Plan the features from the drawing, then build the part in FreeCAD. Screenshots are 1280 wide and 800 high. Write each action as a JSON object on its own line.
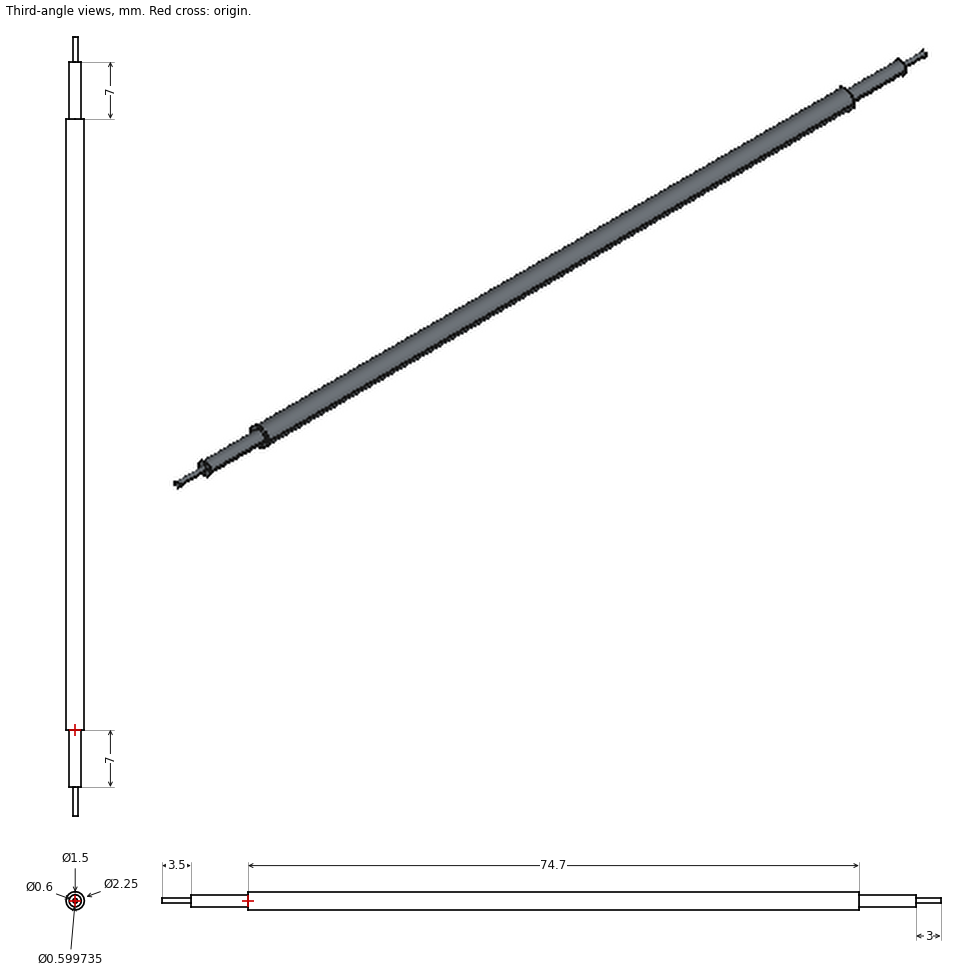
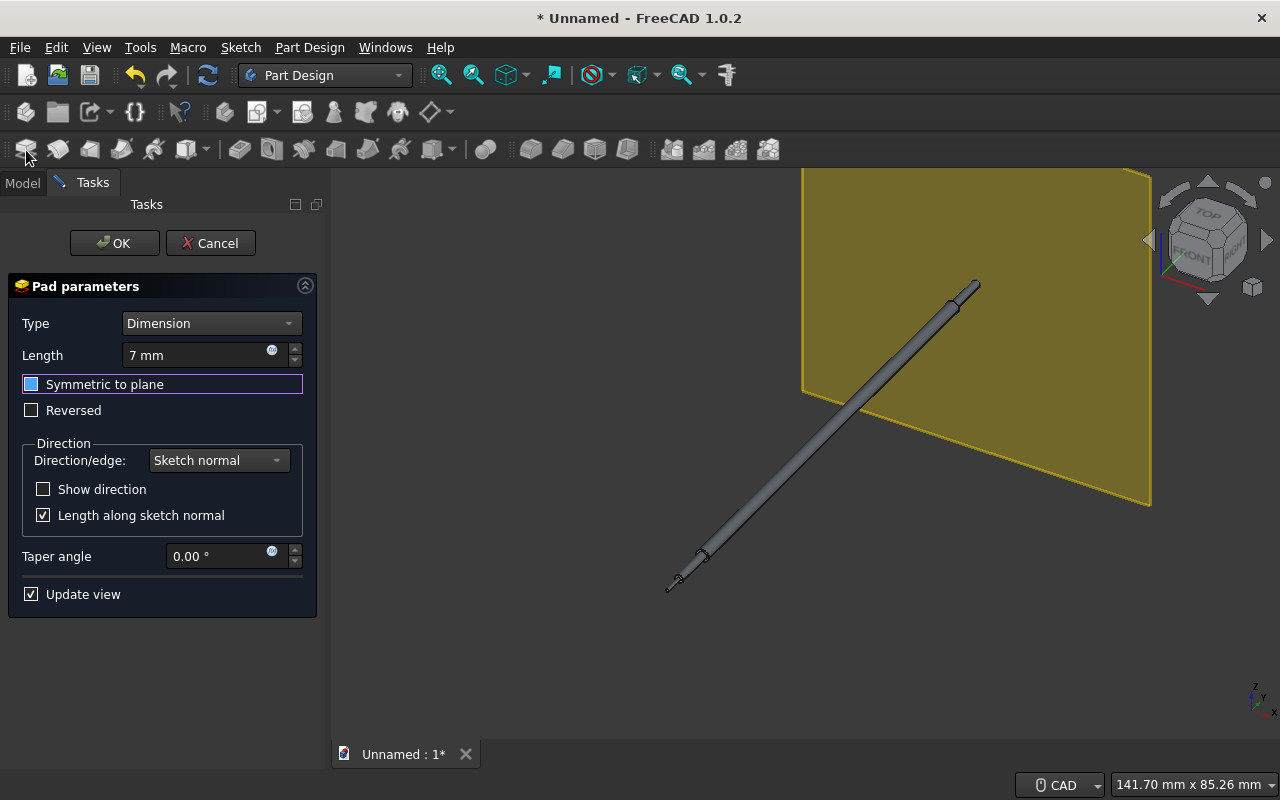
{"action": "left_click", "coordinate": [115, 243]}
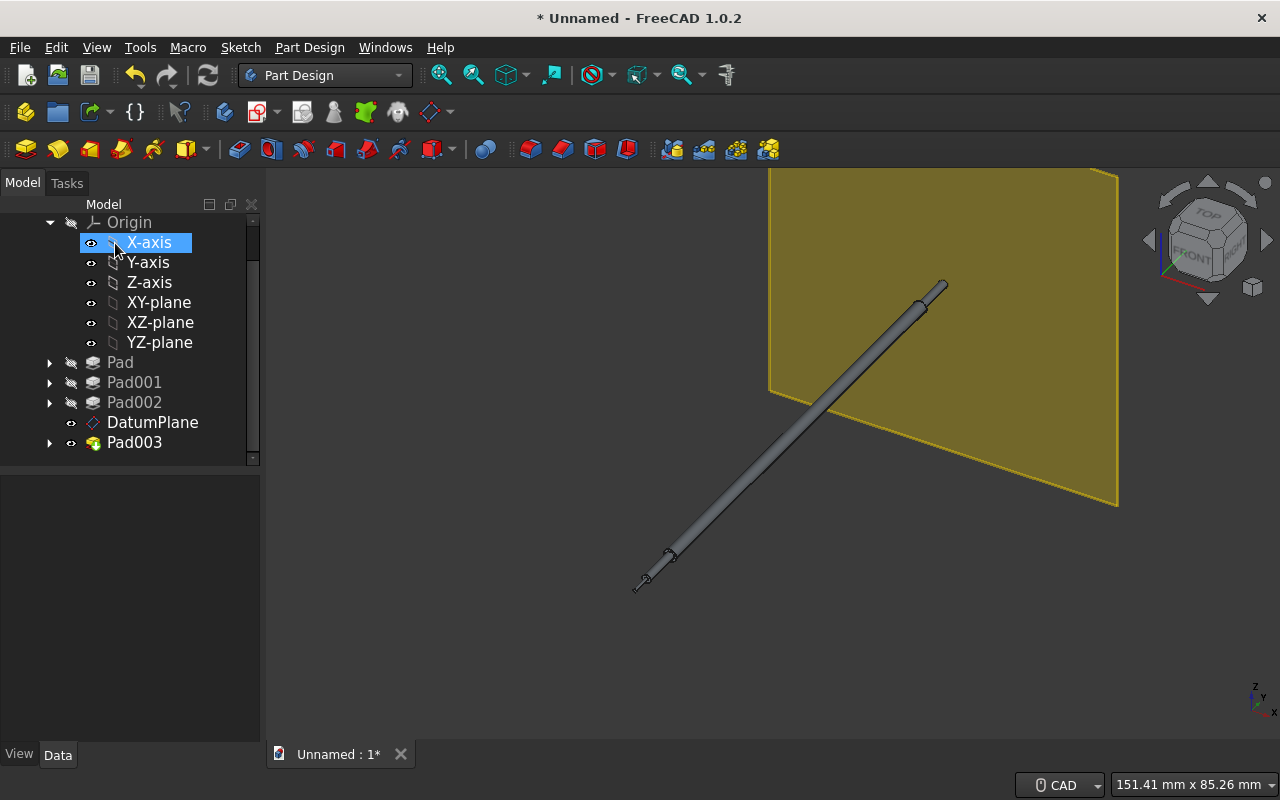
{"action": "left_click", "coordinate": [116, 423]}
{"action": "key", "text": "space"}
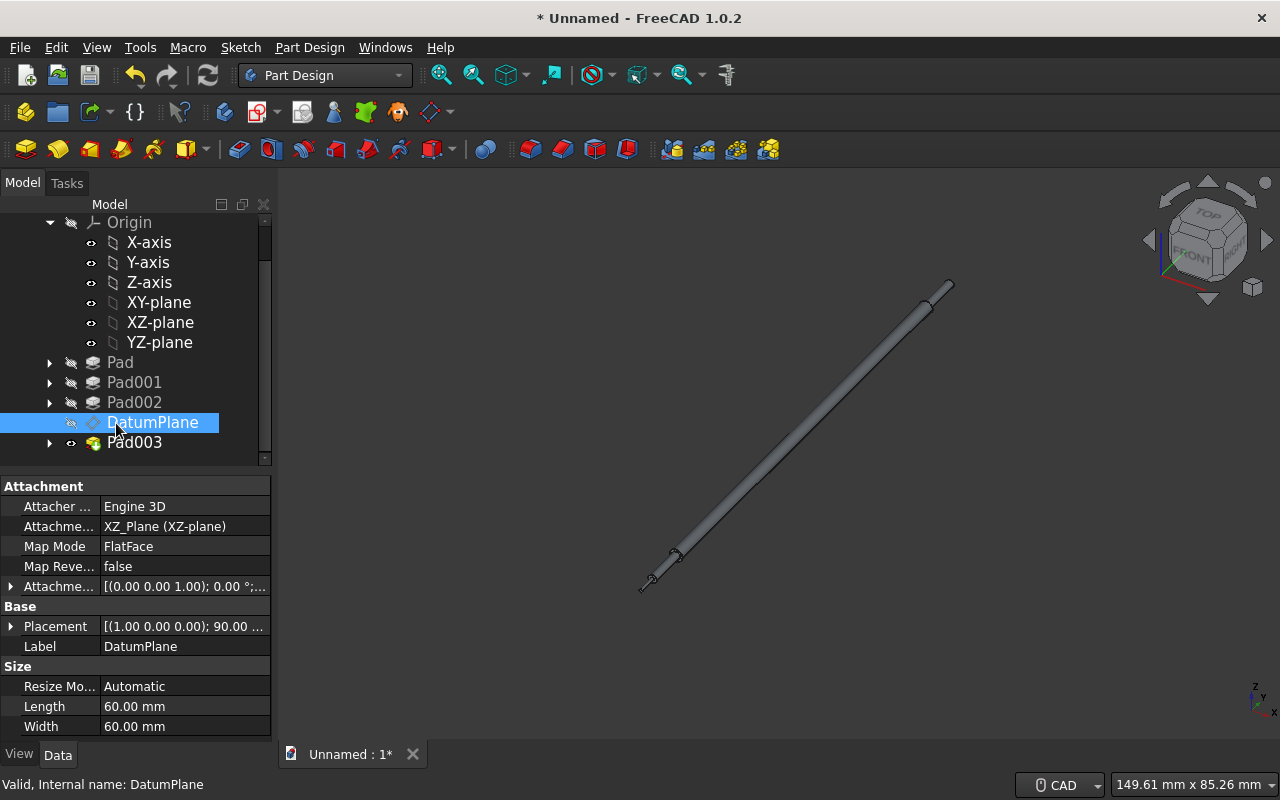
{"action": "key", "text": "4"}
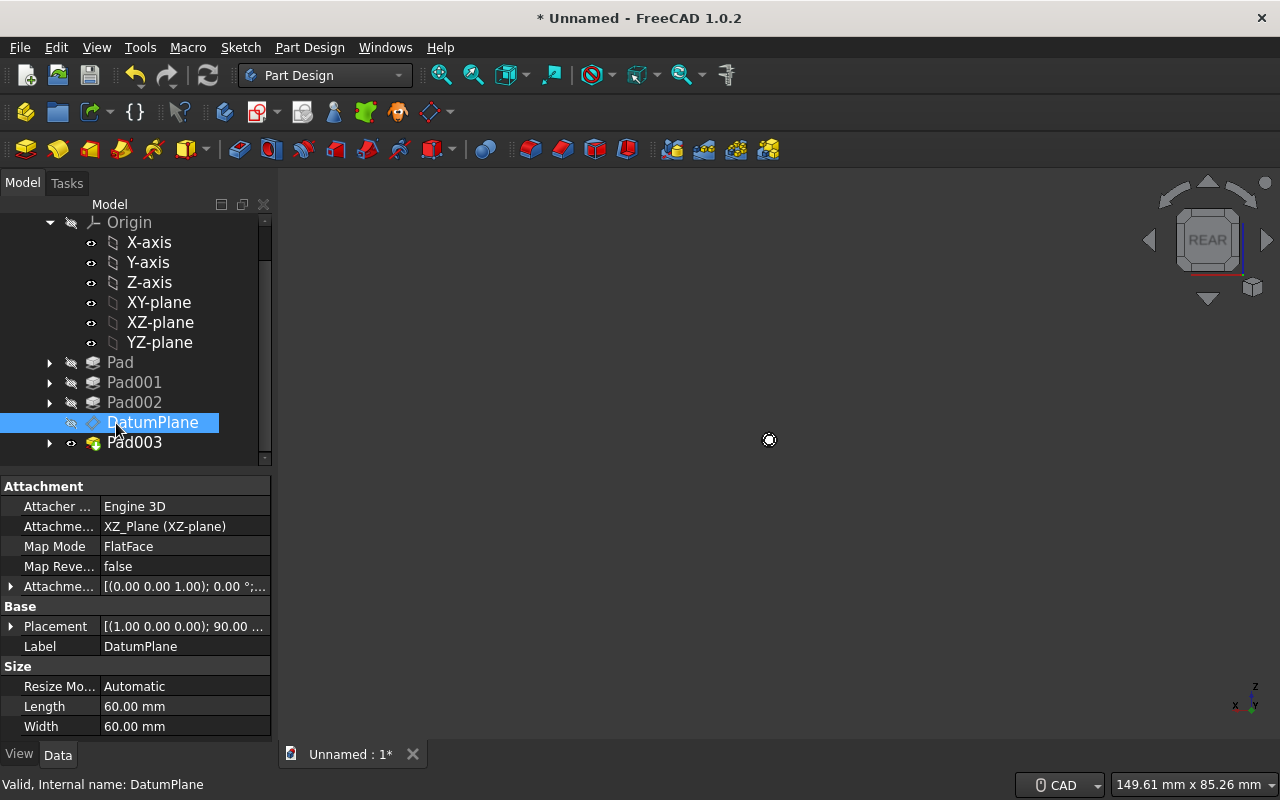
{"action": "left_click", "coordinate": [442, 76]}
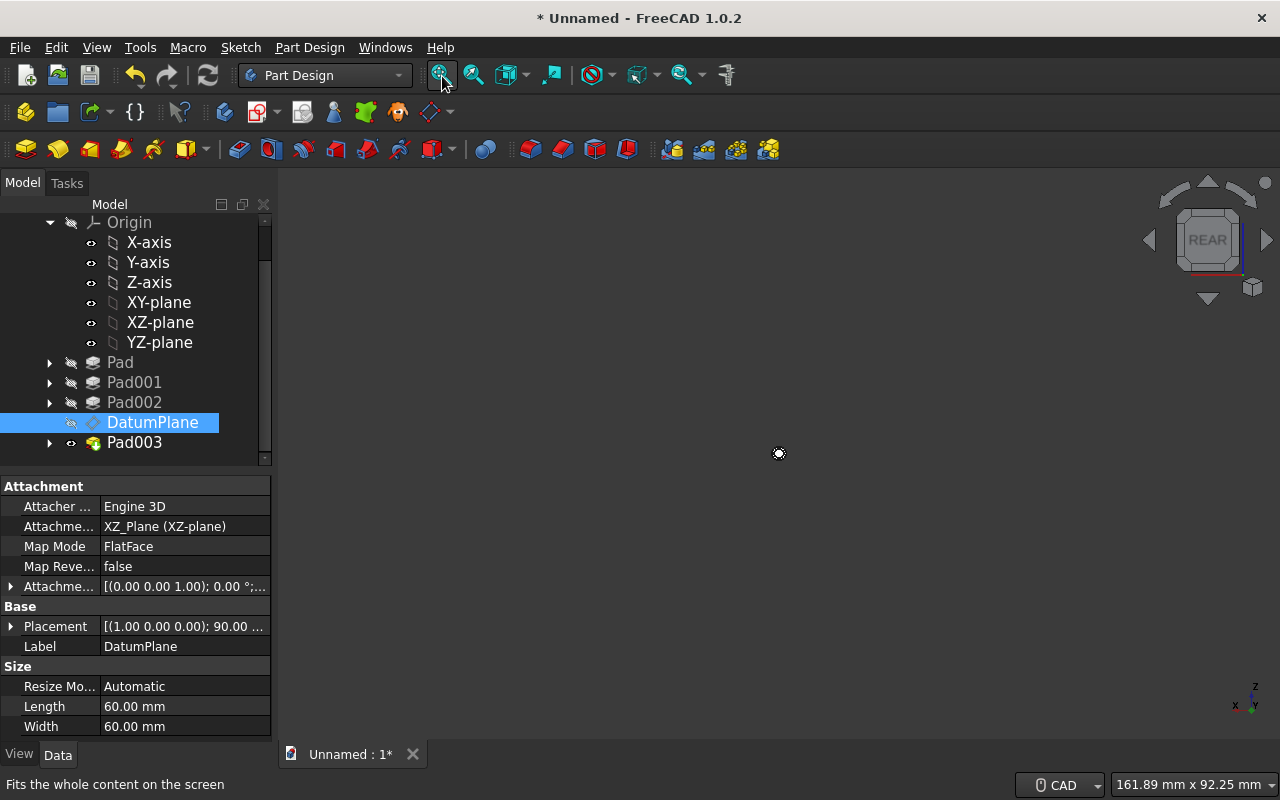
{"action": "scroll", "coordinate": [779, 453], "scroll_direction": "up", "scroll_amount": 5}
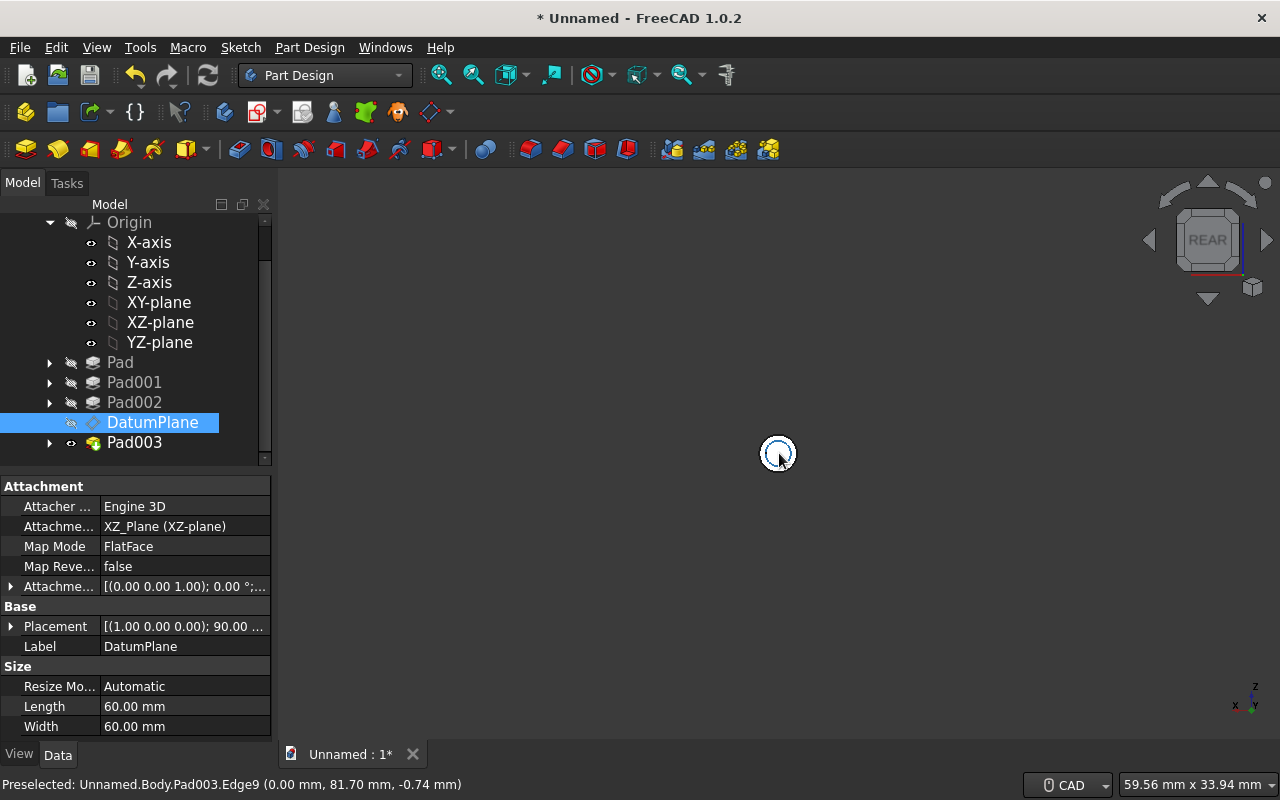
{"action": "left_click", "coordinate": [778, 453]}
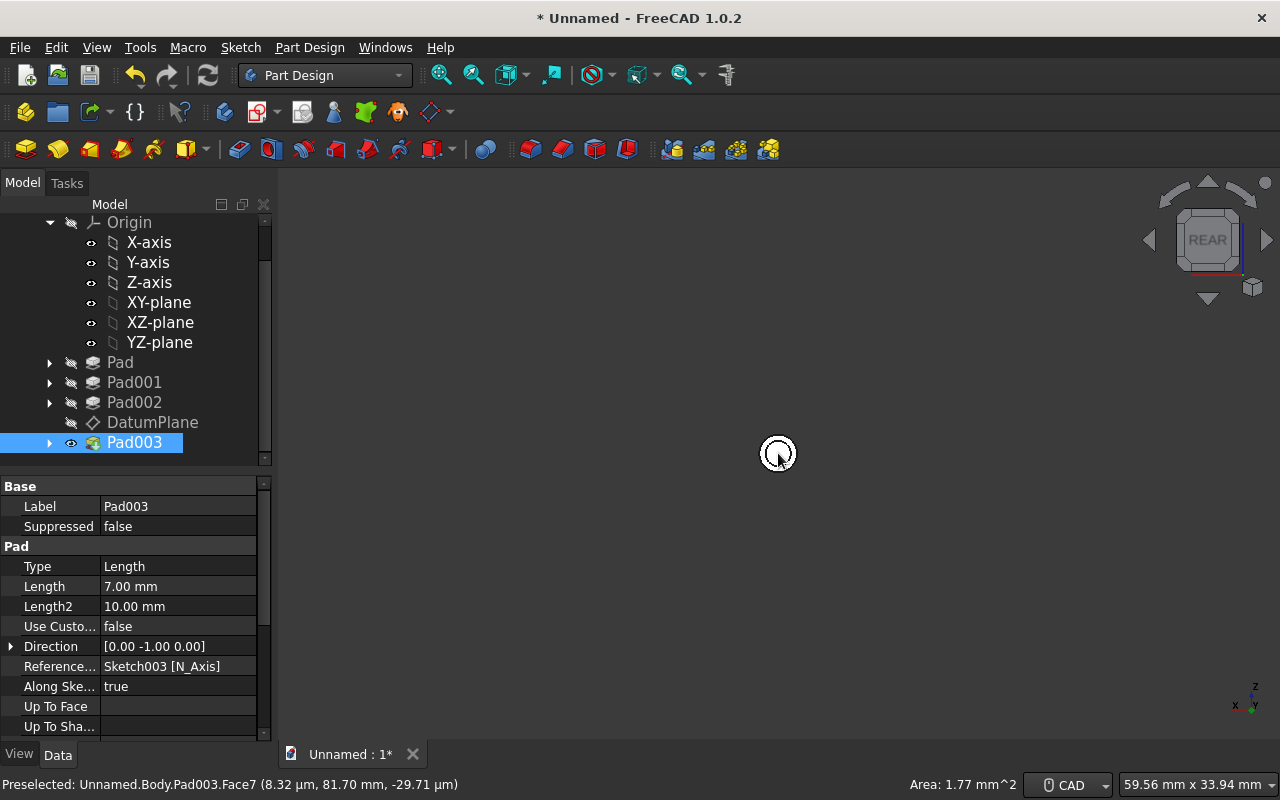
{"action": "left_click", "coordinate": [258, 112]}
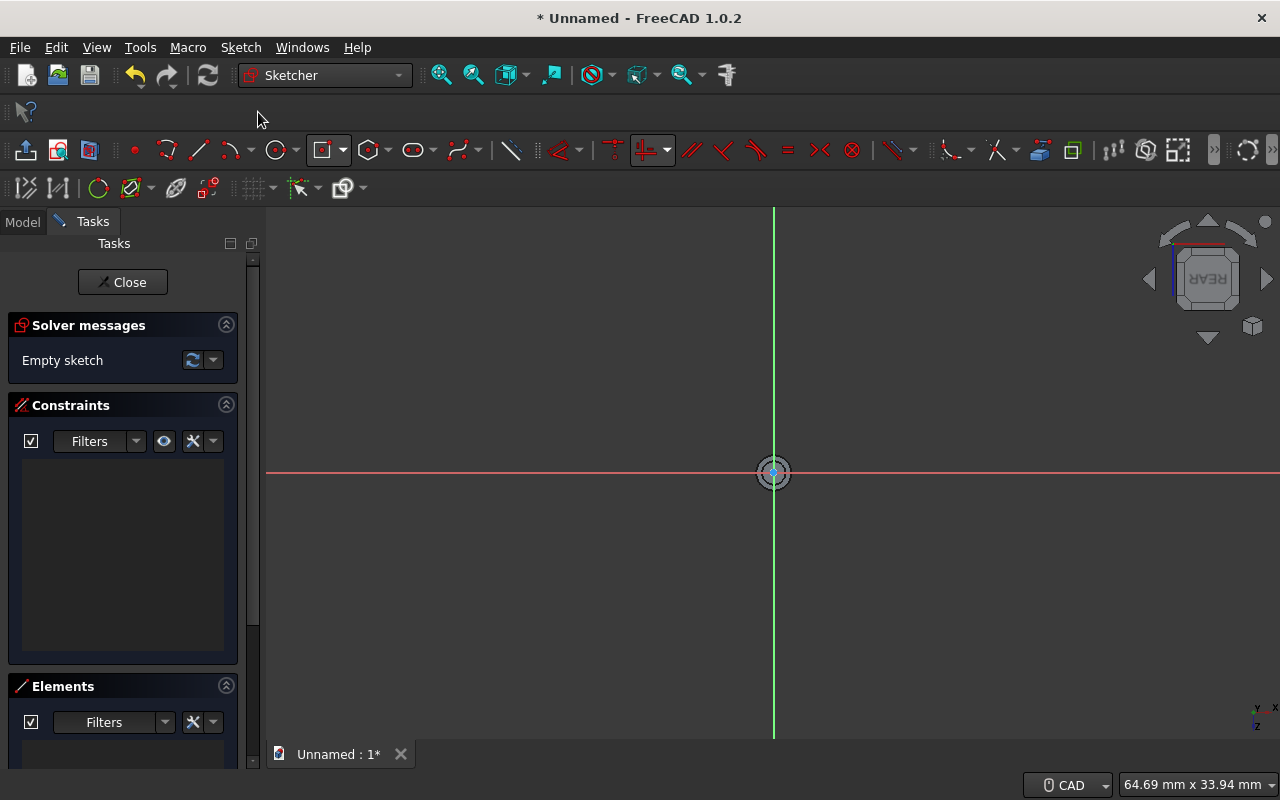
{"action": "scroll", "coordinate": [777, 473], "scroll_direction": "up", "scroll_amount": 15}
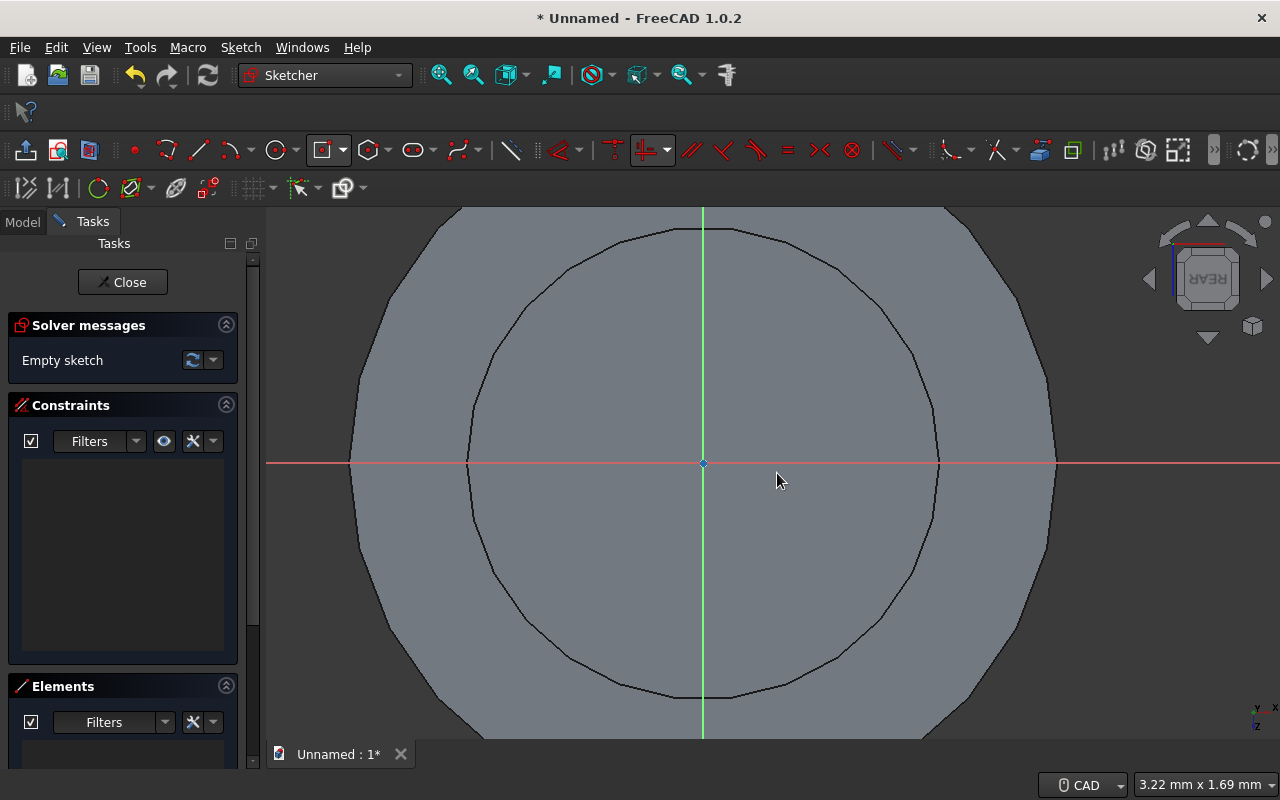
{"action": "scroll", "coordinate": [701, 452], "scroll_direction": "up", "scroll_amount": 3}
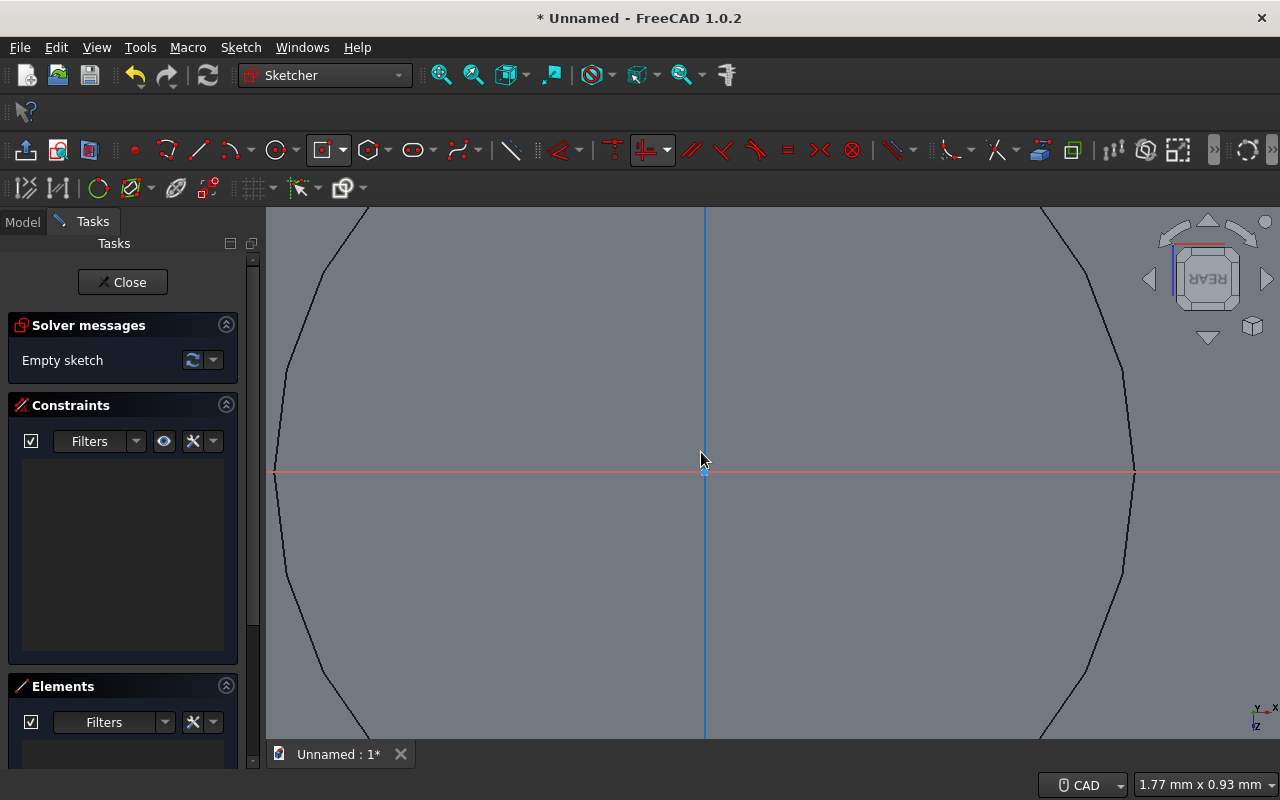
{"action": "left_click", "coordinate": [276, 150]}